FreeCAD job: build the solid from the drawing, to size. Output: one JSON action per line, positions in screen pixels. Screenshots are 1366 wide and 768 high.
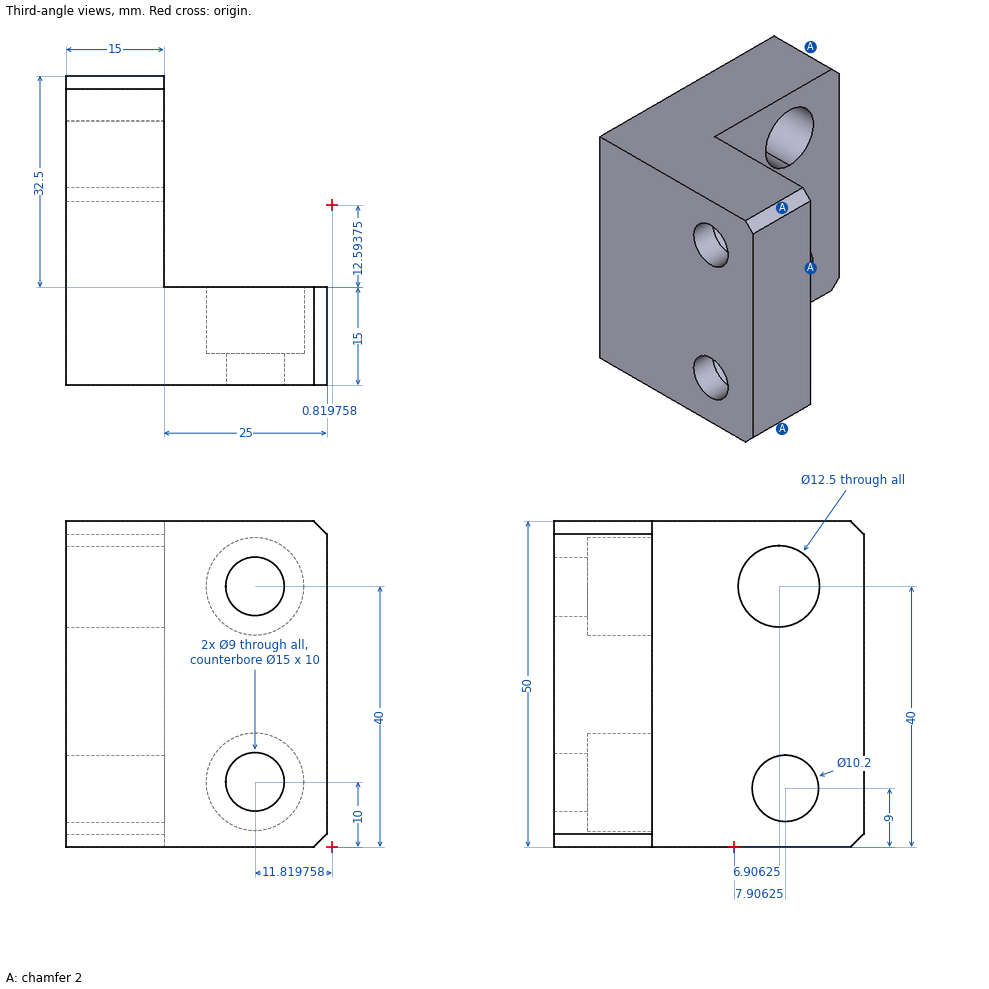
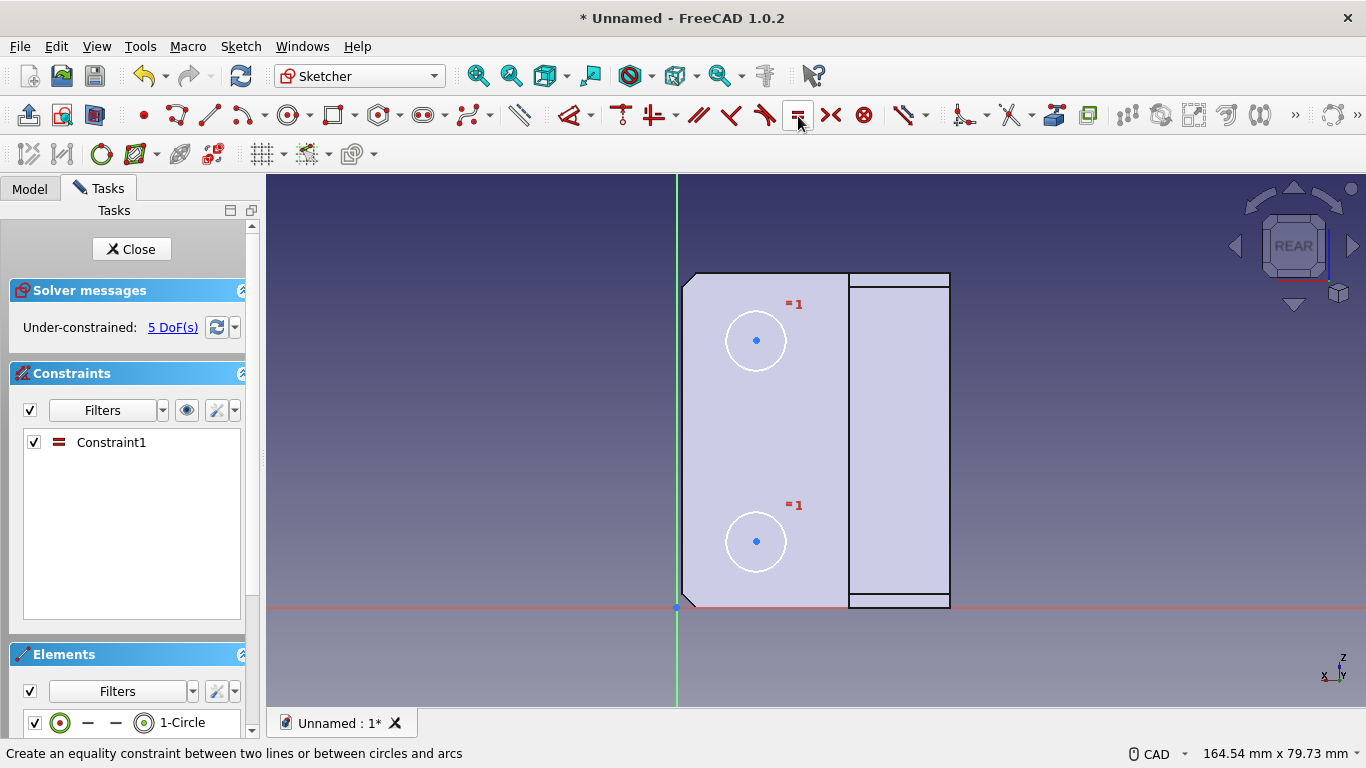
{"action": "left_click", "coordinate": [756, 542]}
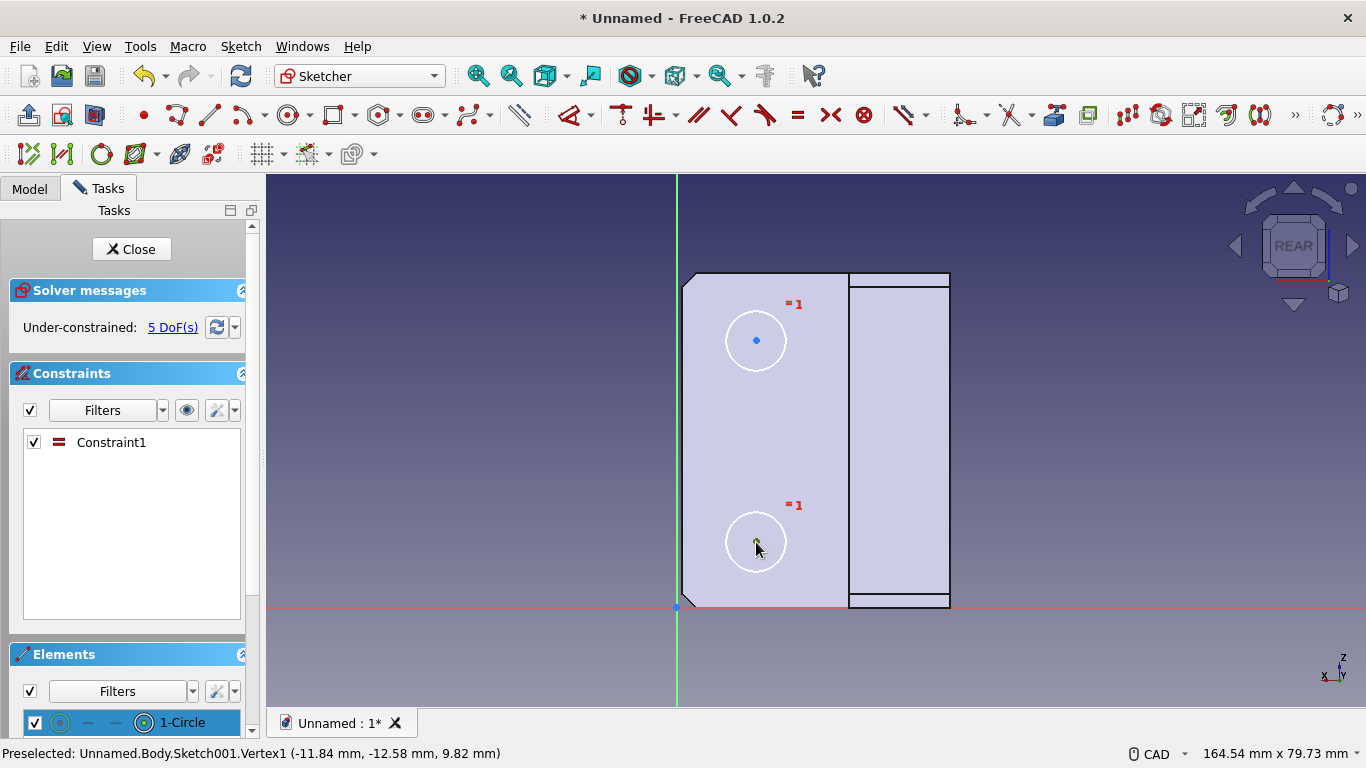
{"action": "left_click", "coordinate": [756, 341]}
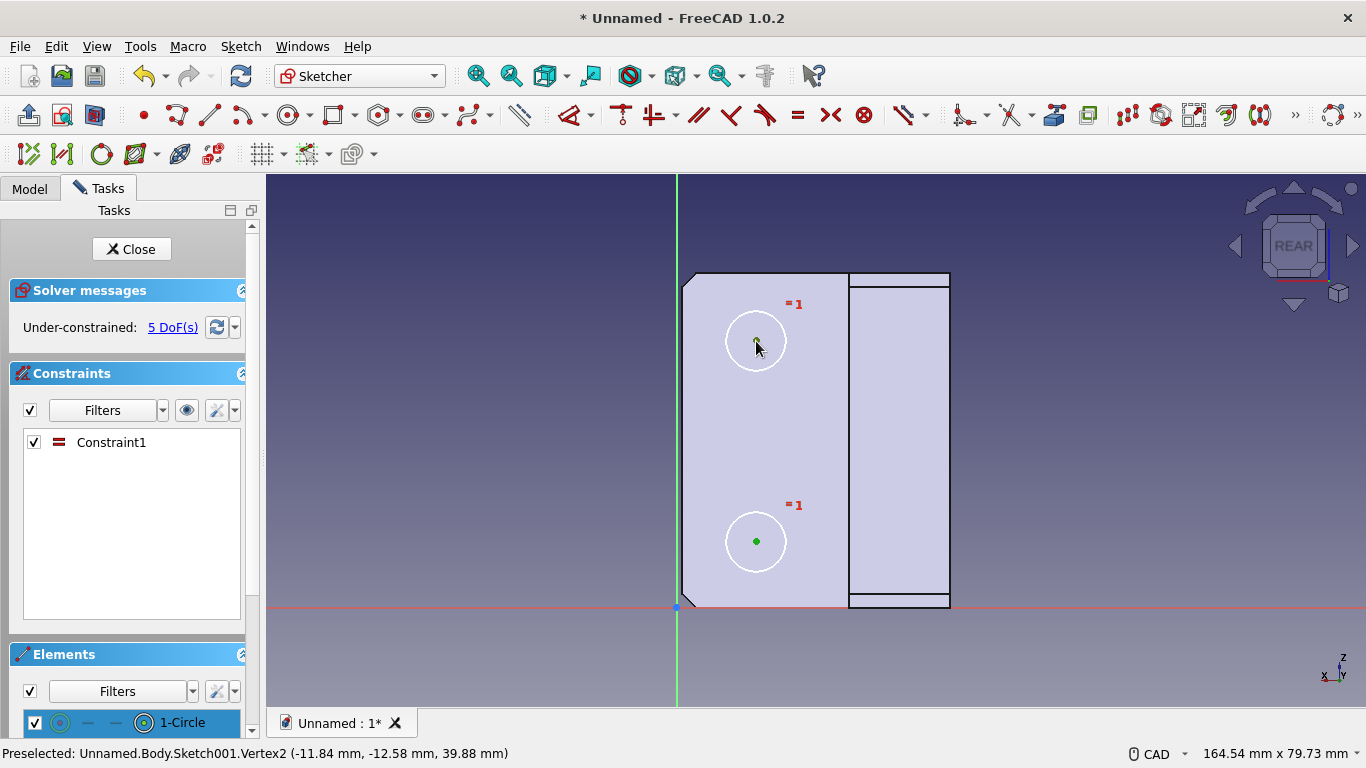
{"action": "key", "text": "v"}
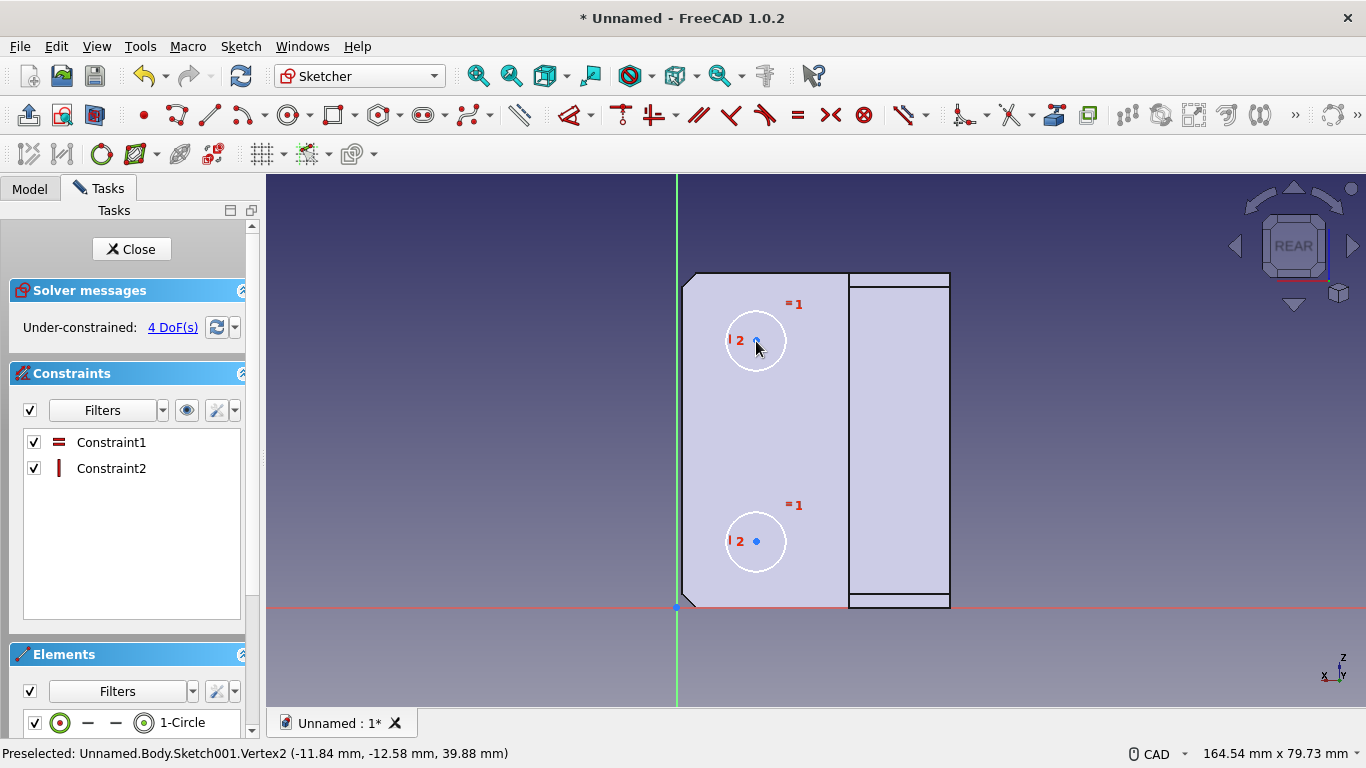
{"action": "left_click", "coordinate": [568, 116]}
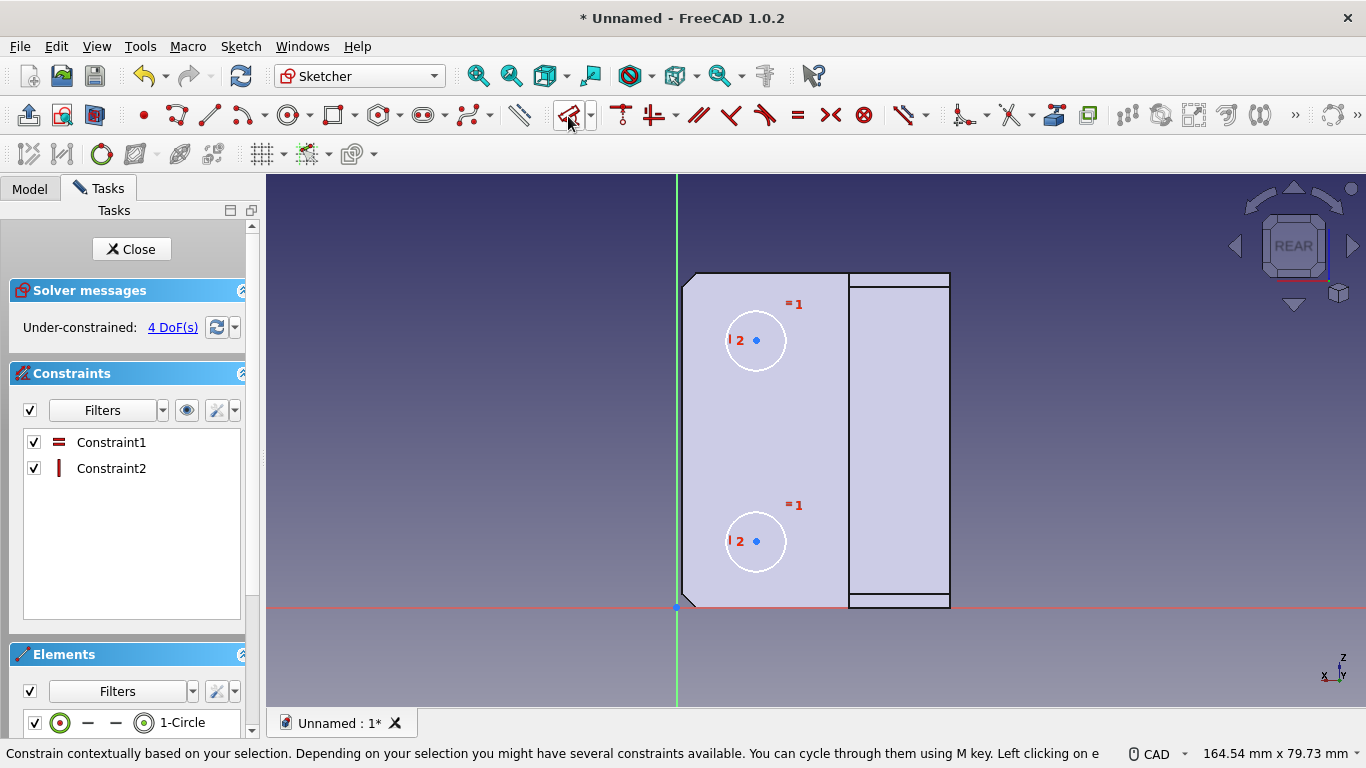
{"action": "left_click", "coordinate": [777, 521]}
{"action": "left_click", "coordinate": [800, 498]}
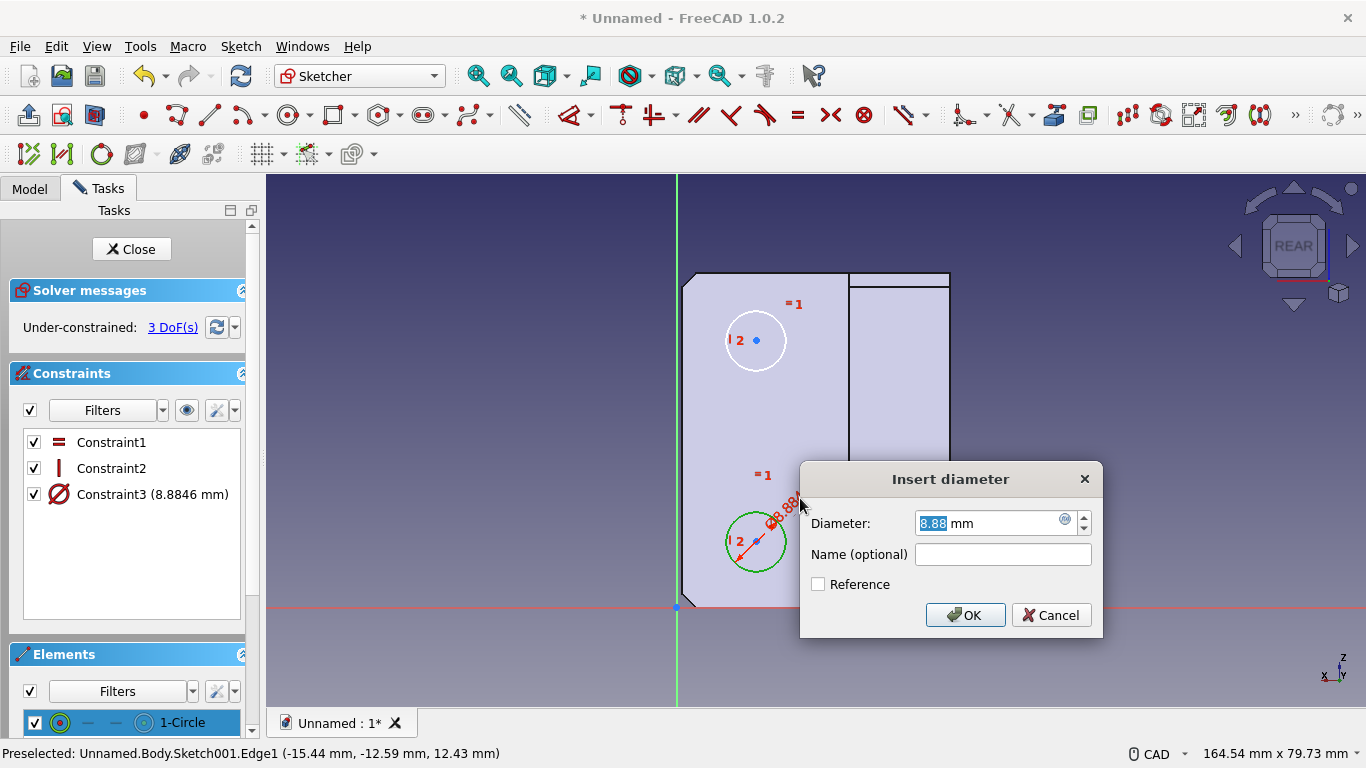
{"action": "type", "text": "9"}
{"action": "key", "text": "Return"}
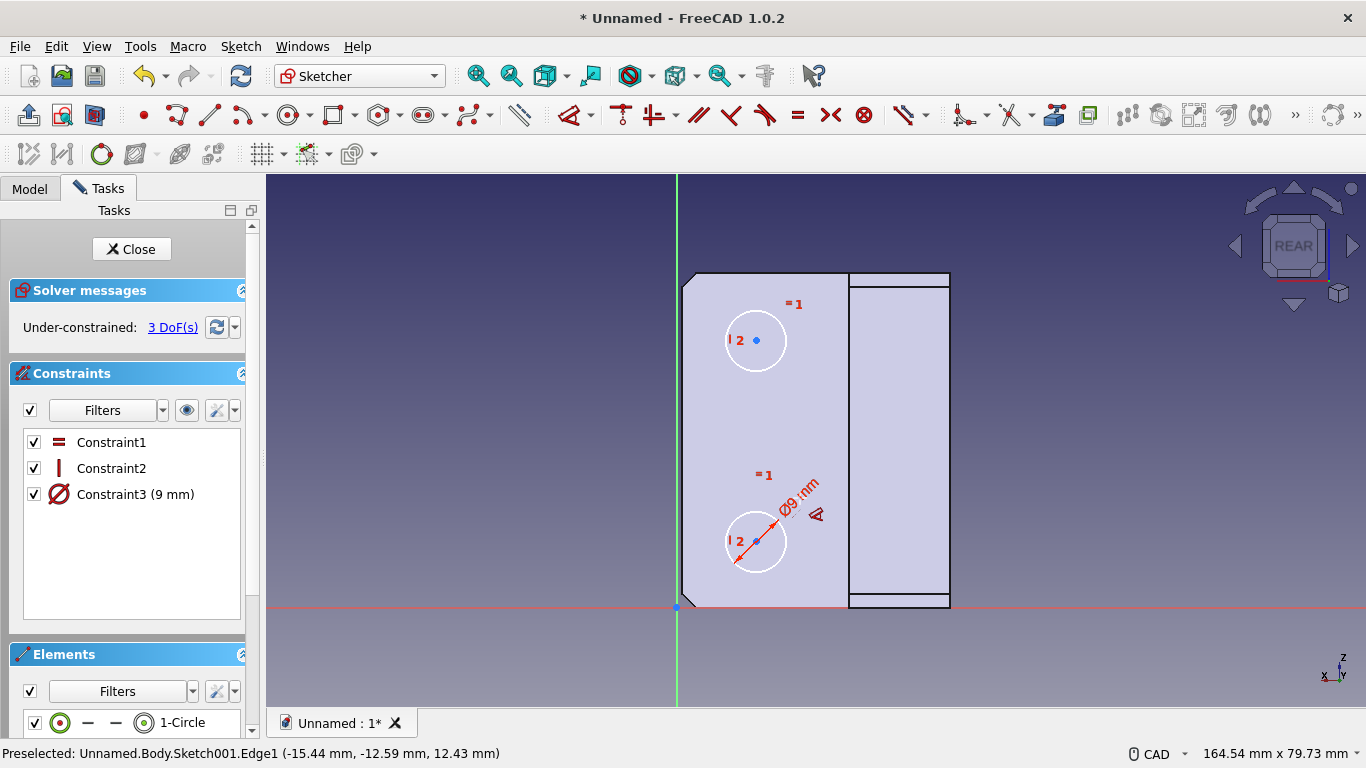
{"action": "left_click", "coordinate": [756, 542]}
{"action": "left_click", "coordinate": [643, 575]}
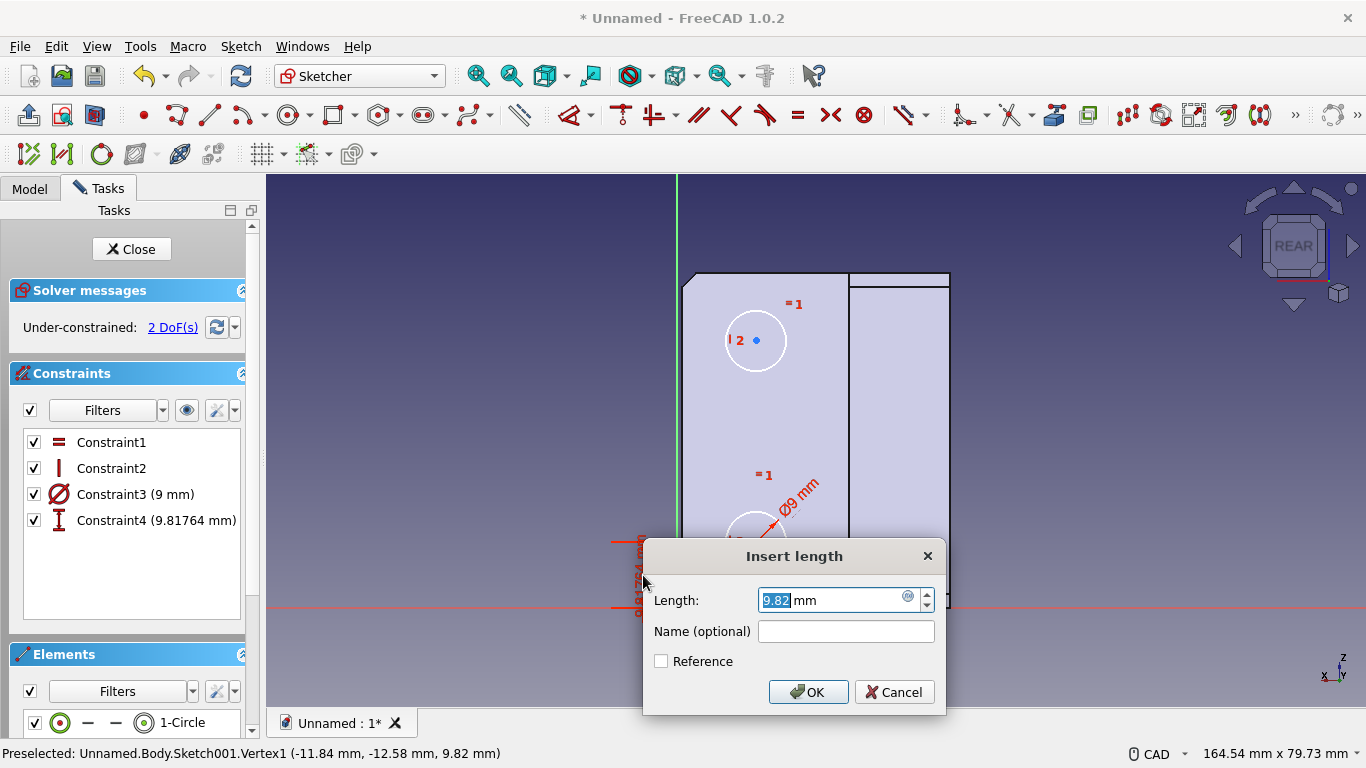
{"action": "type", "text": "10"}
{"action": "key", "text": "Return"}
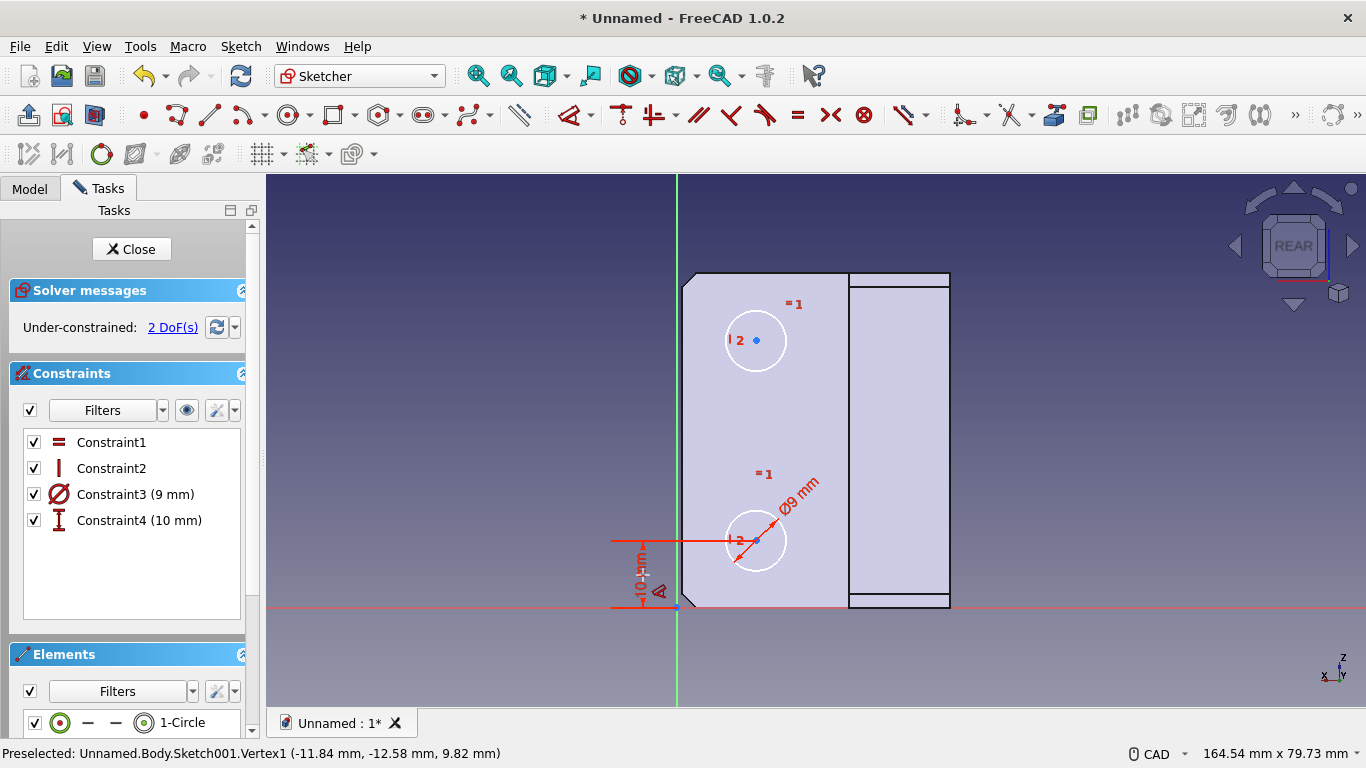
{"action": "left_click", "coordinate": [756, 341]}
{"action": "left_click", "coordinate": [643, 474]}